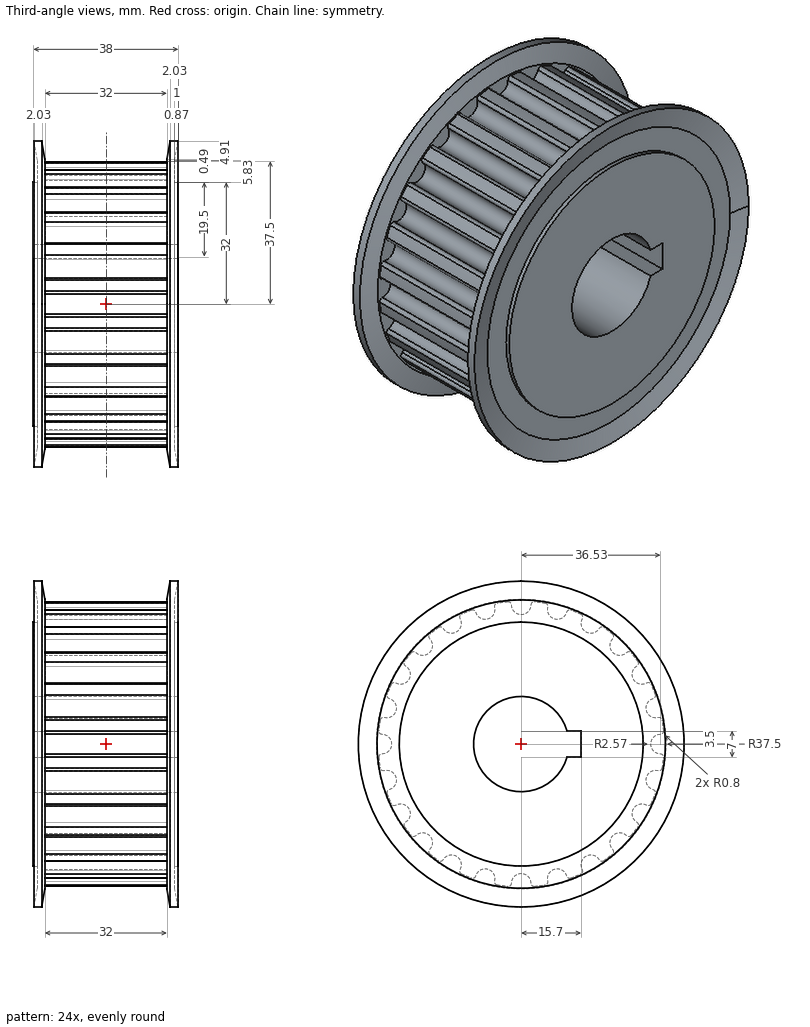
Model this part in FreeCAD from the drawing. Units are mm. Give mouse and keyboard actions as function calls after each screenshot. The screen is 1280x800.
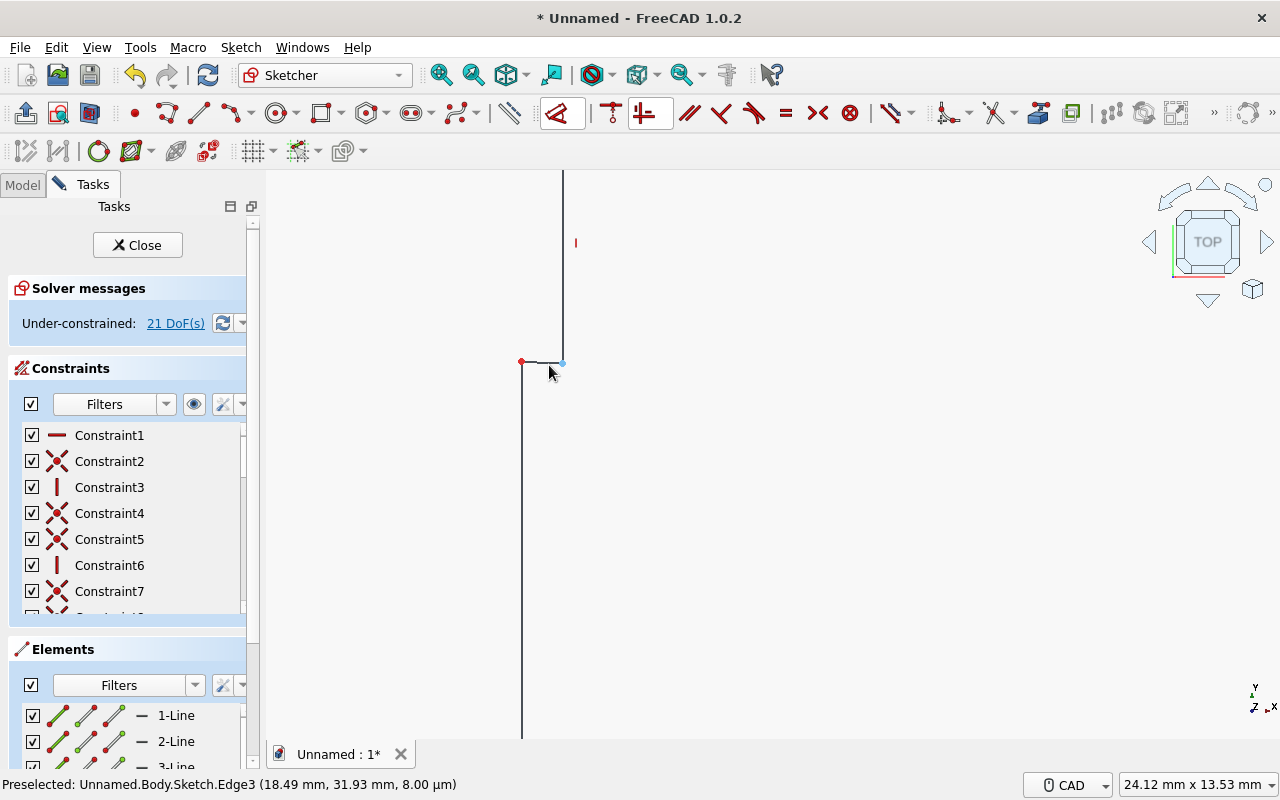
click(546, 363)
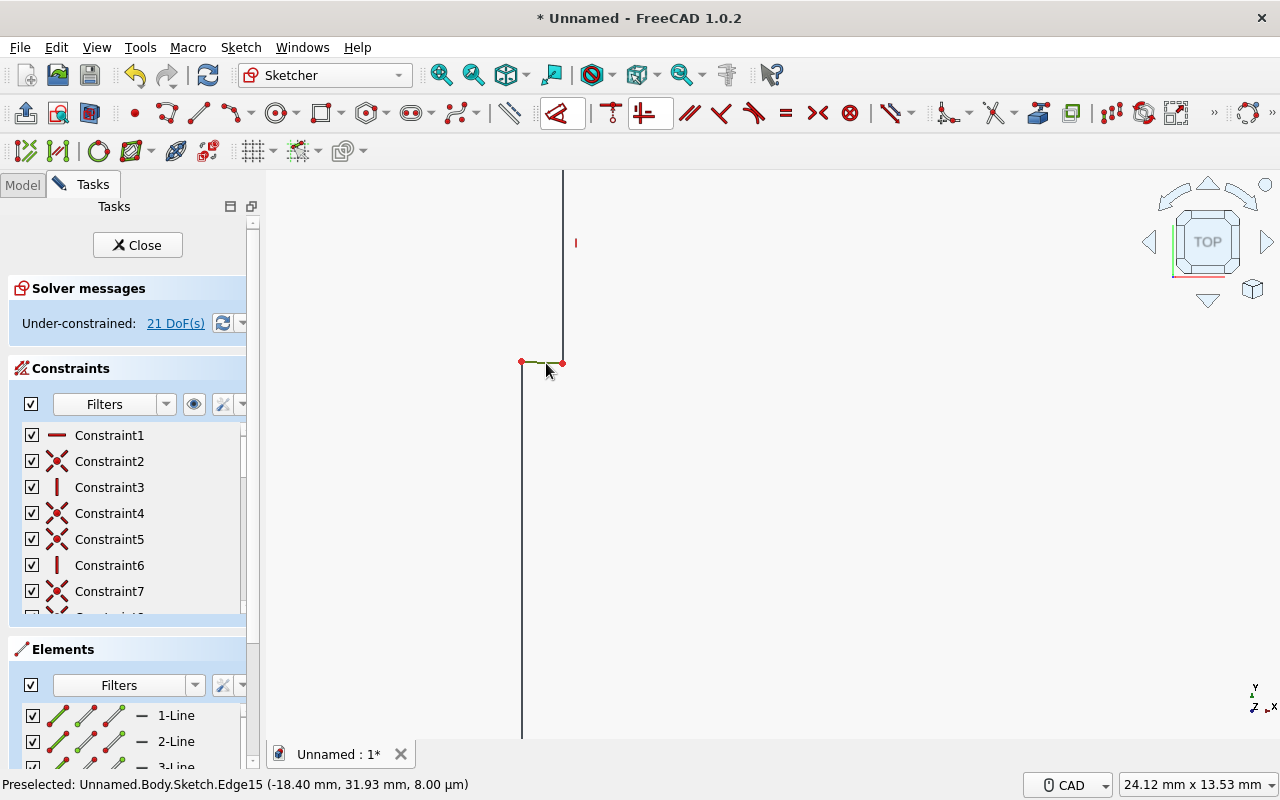
key(h)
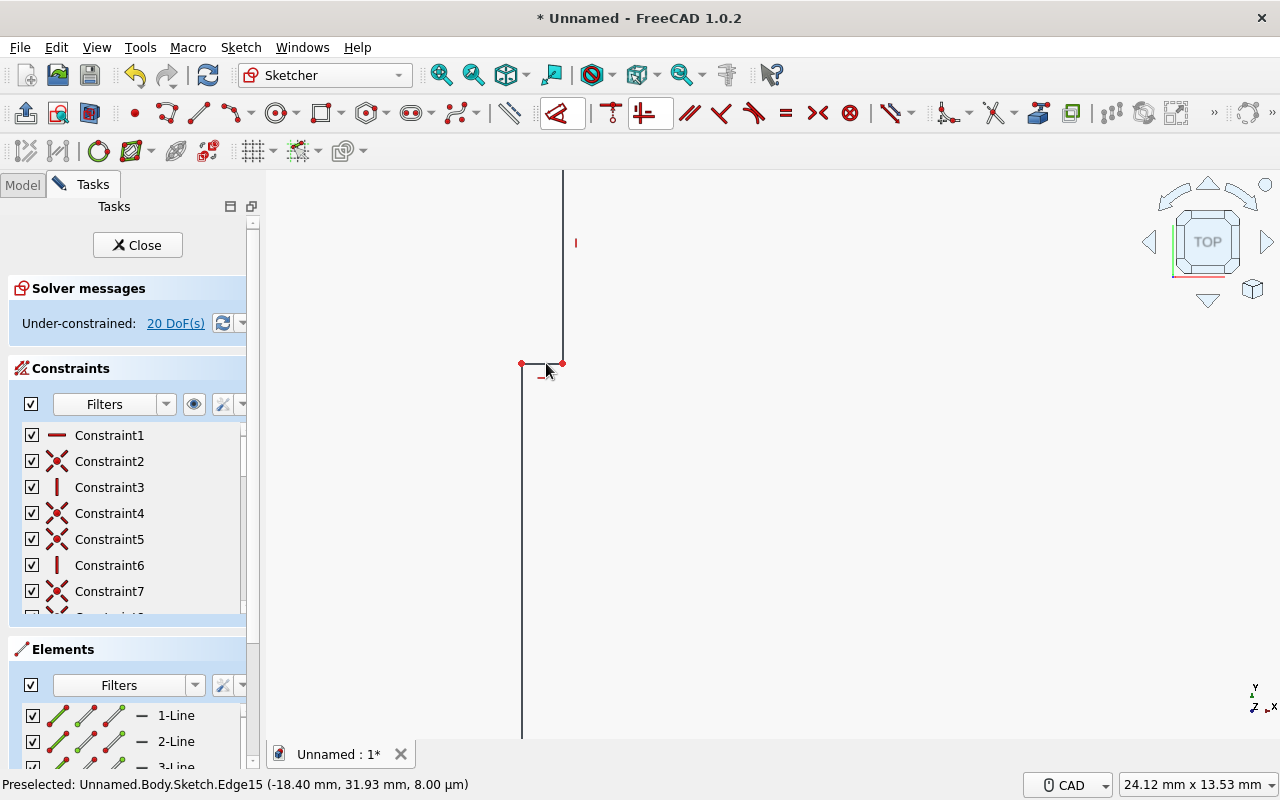
scroll(549, 365, down, 8)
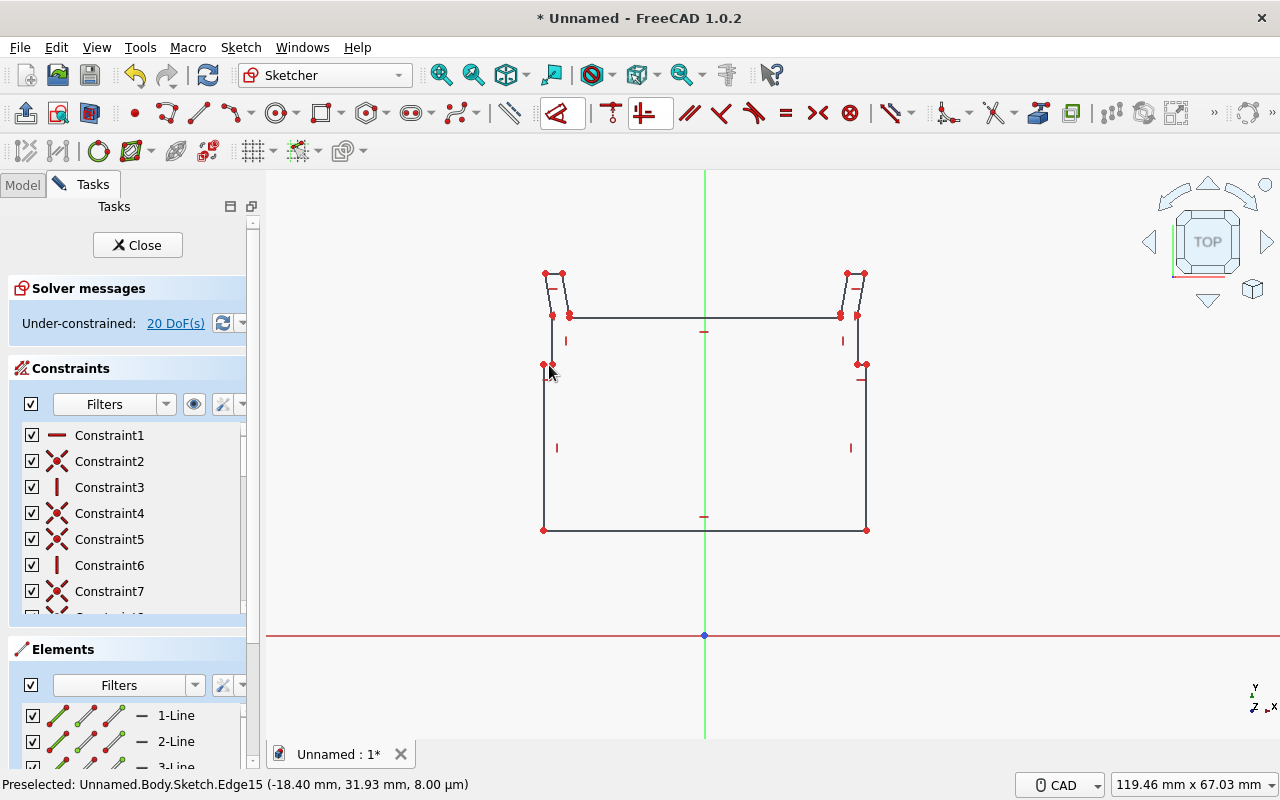
scroll(841, 314, up, 6)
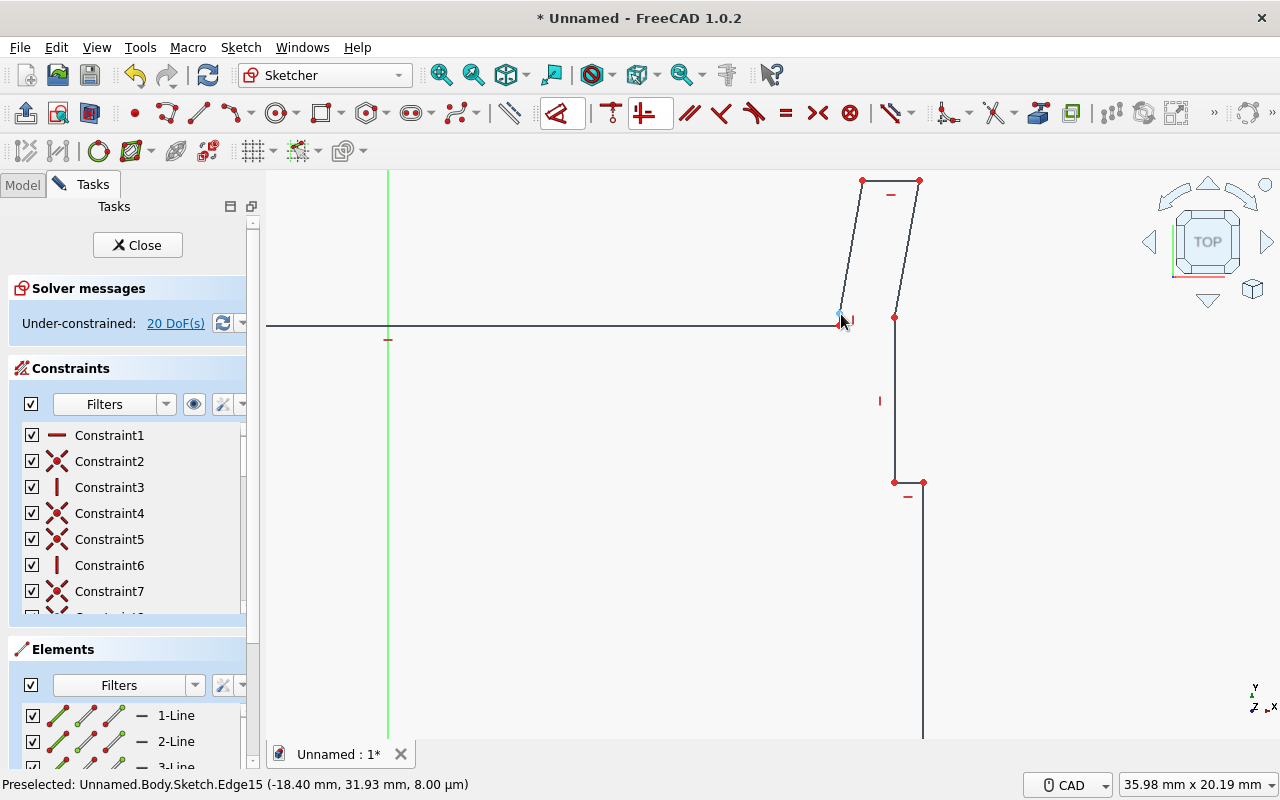
click(840, 313)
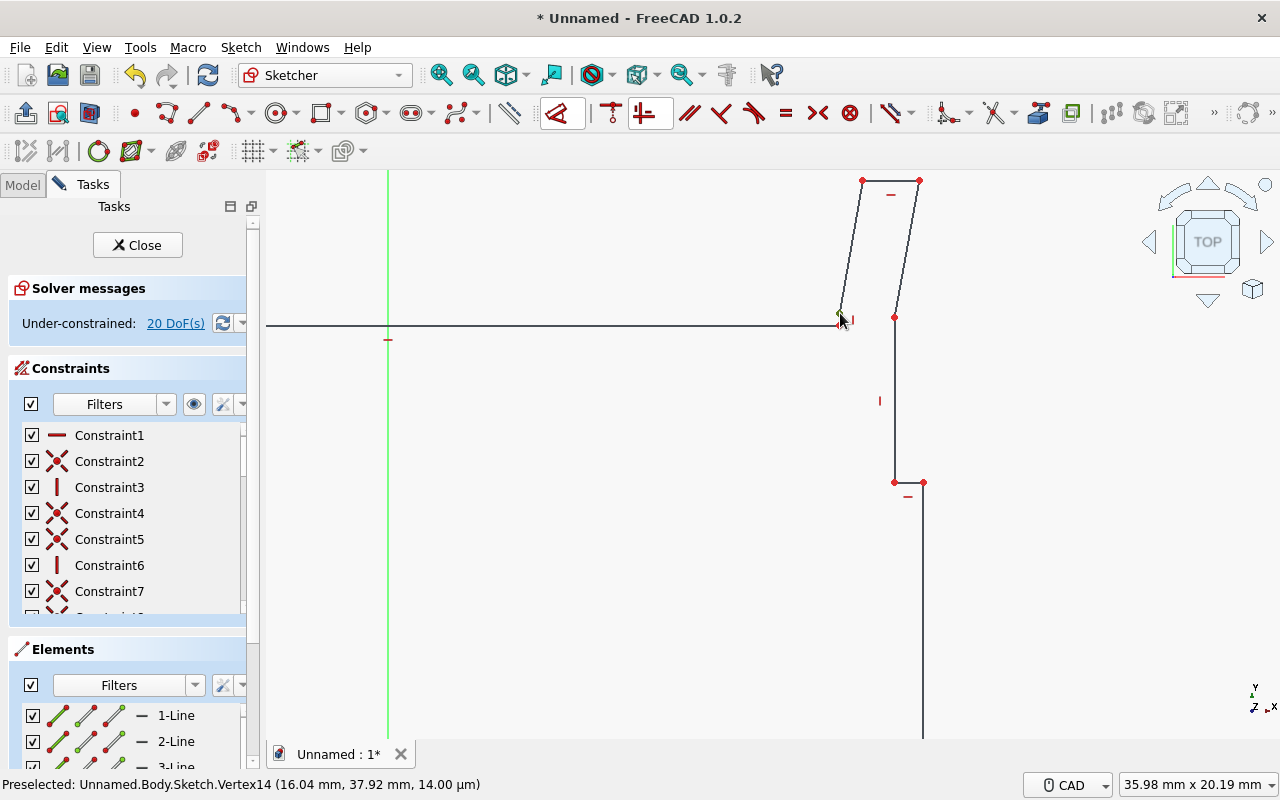
scroll(841, 314, down, 6)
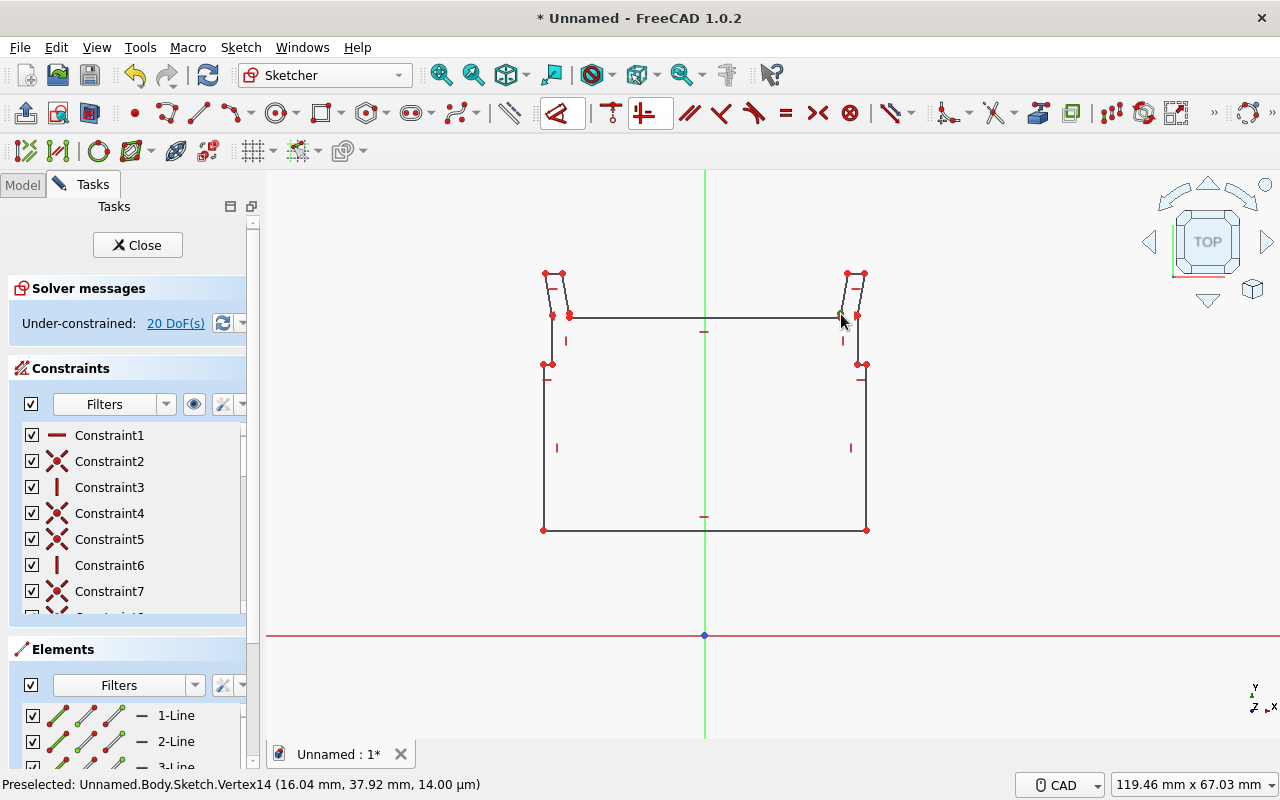
scroll(569, 314, up, 6)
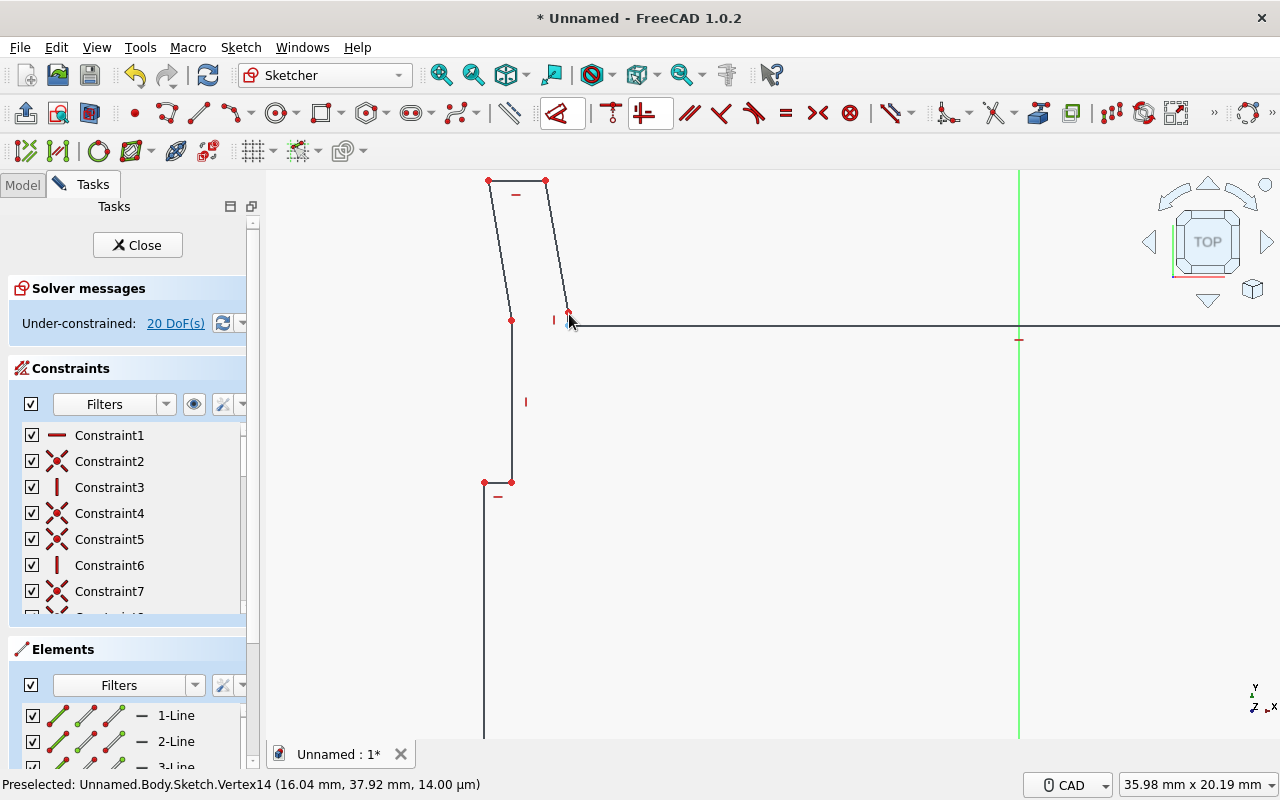
click(568, 312)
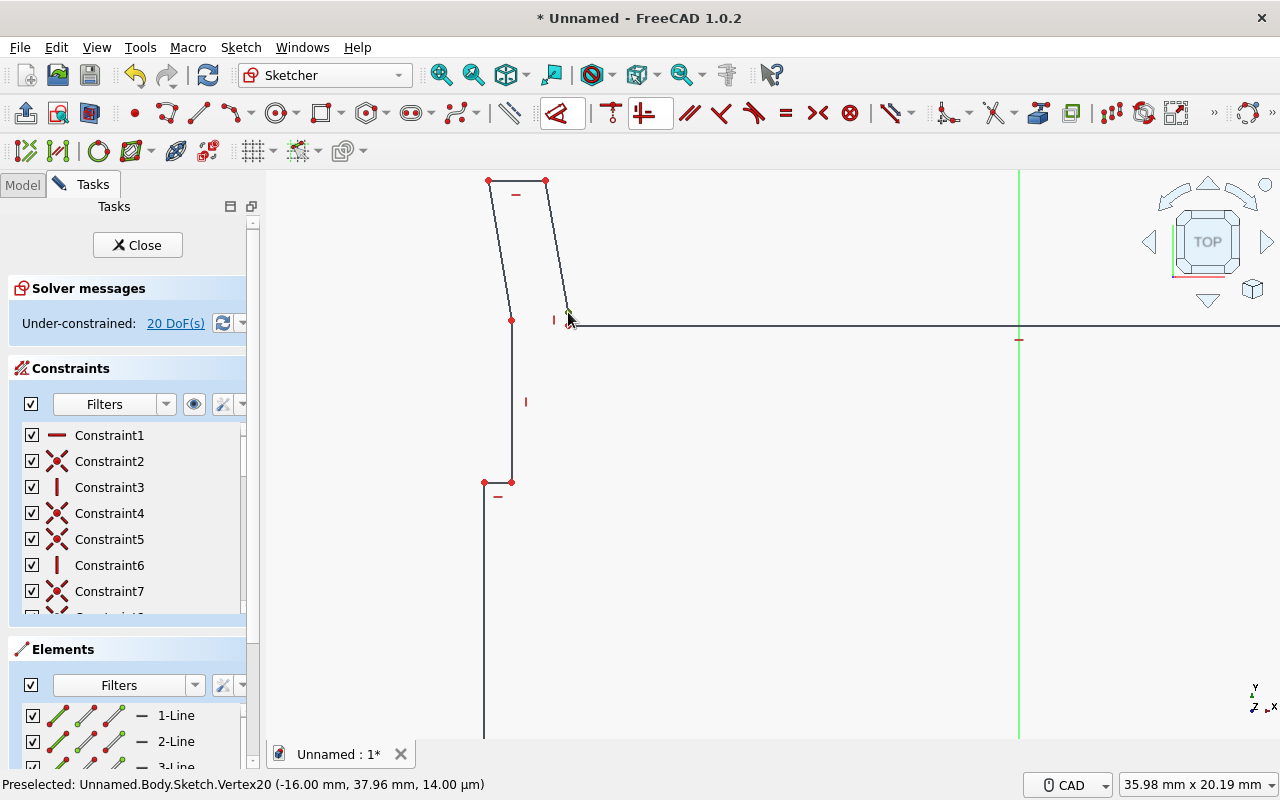
click(1019, 674)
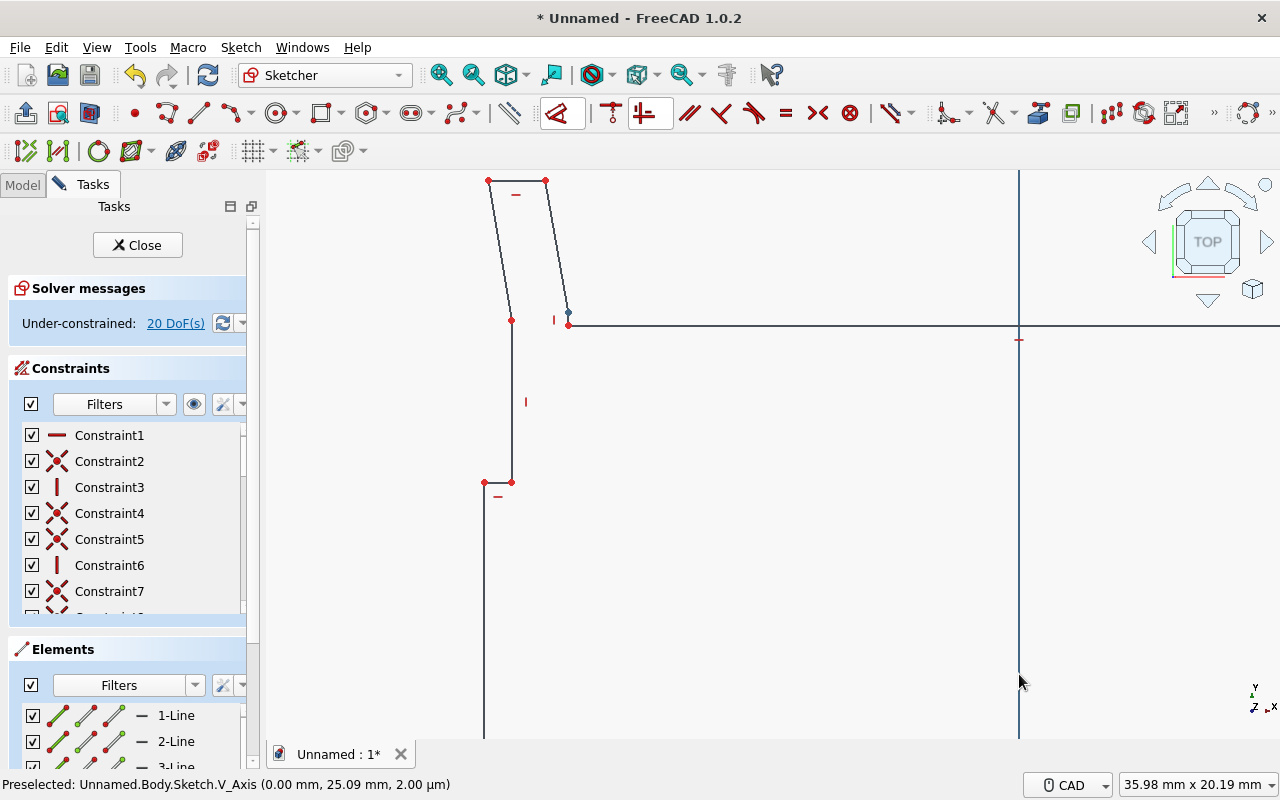
click(818, 114)